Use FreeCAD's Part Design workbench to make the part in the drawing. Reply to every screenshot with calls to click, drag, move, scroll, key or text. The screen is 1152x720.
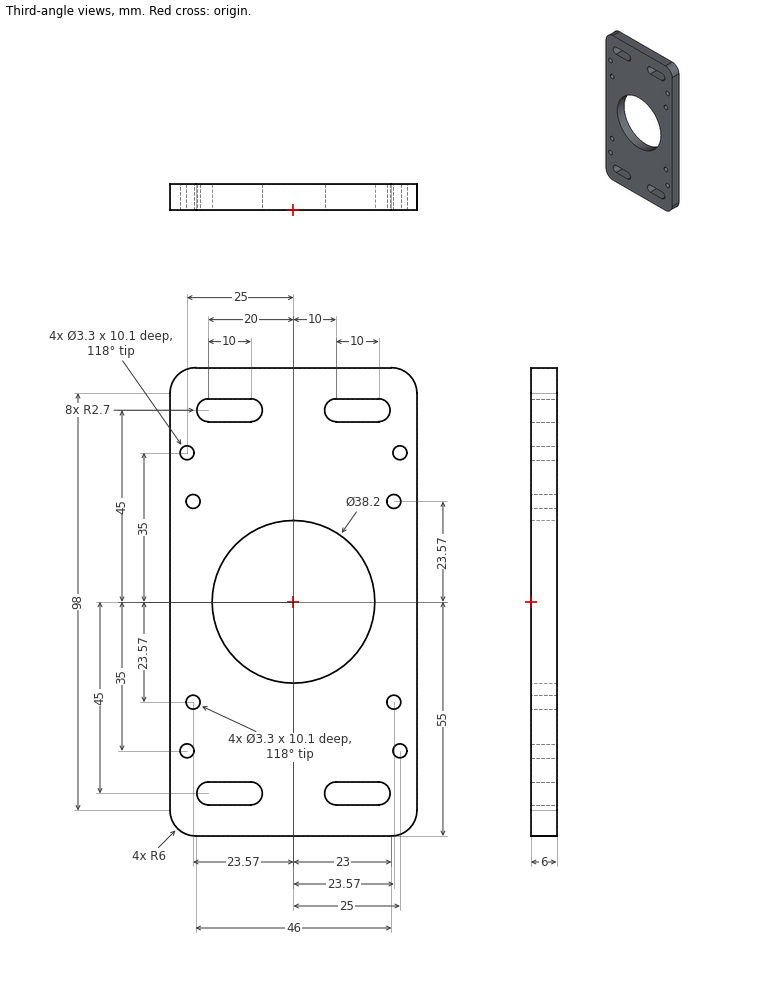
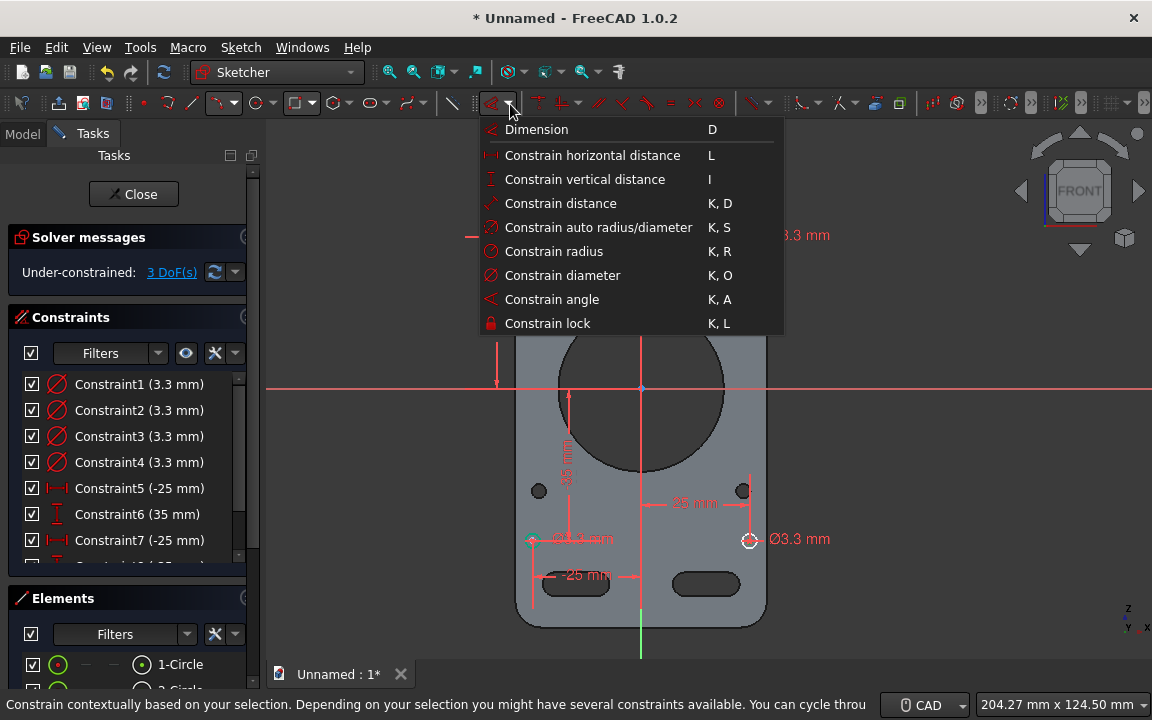
click(632, 179)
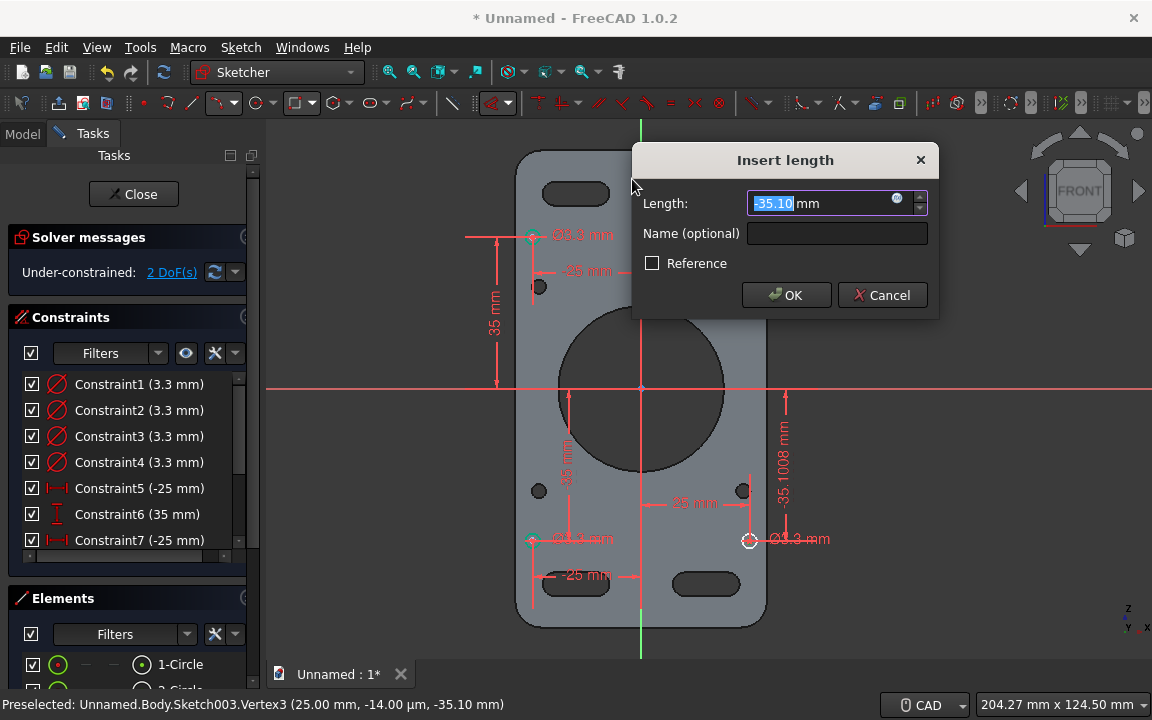
text(-35)
key(Return)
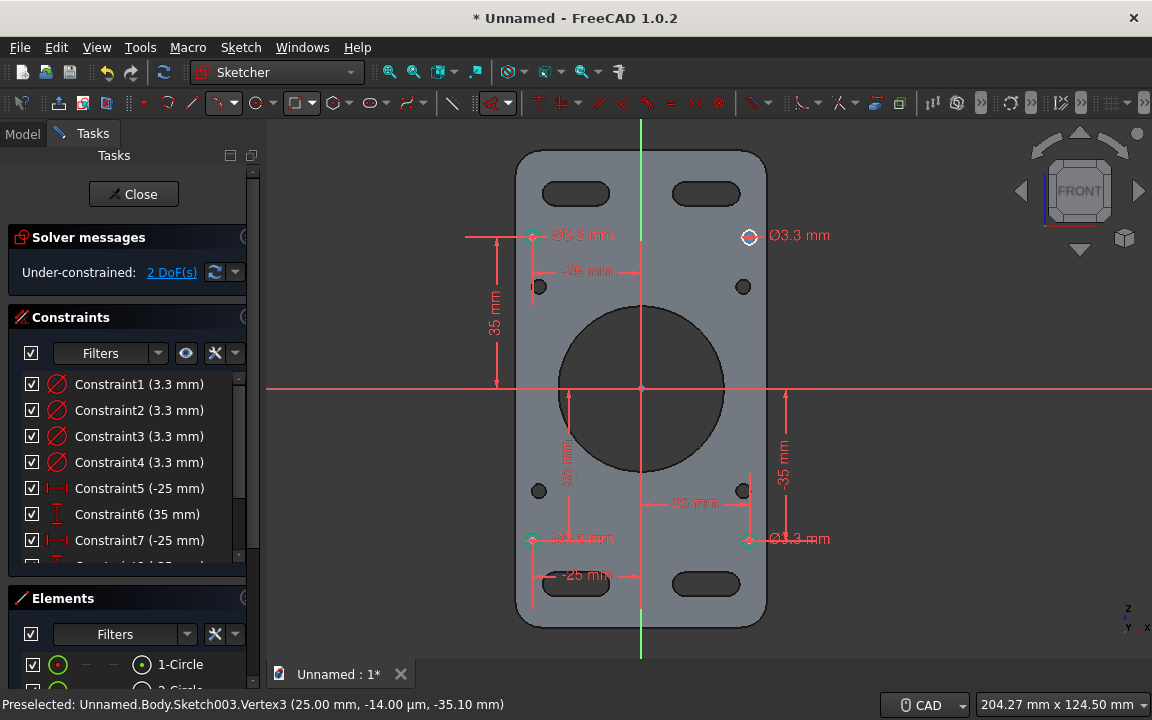
click(749, 237)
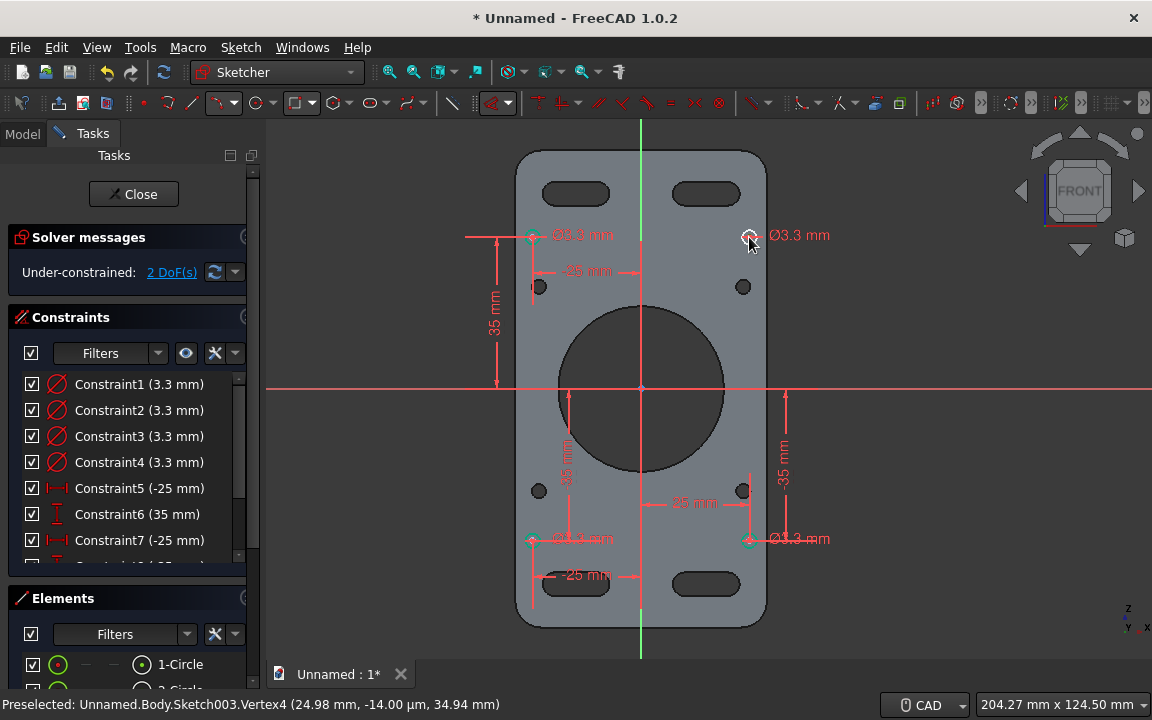
click(510, 104)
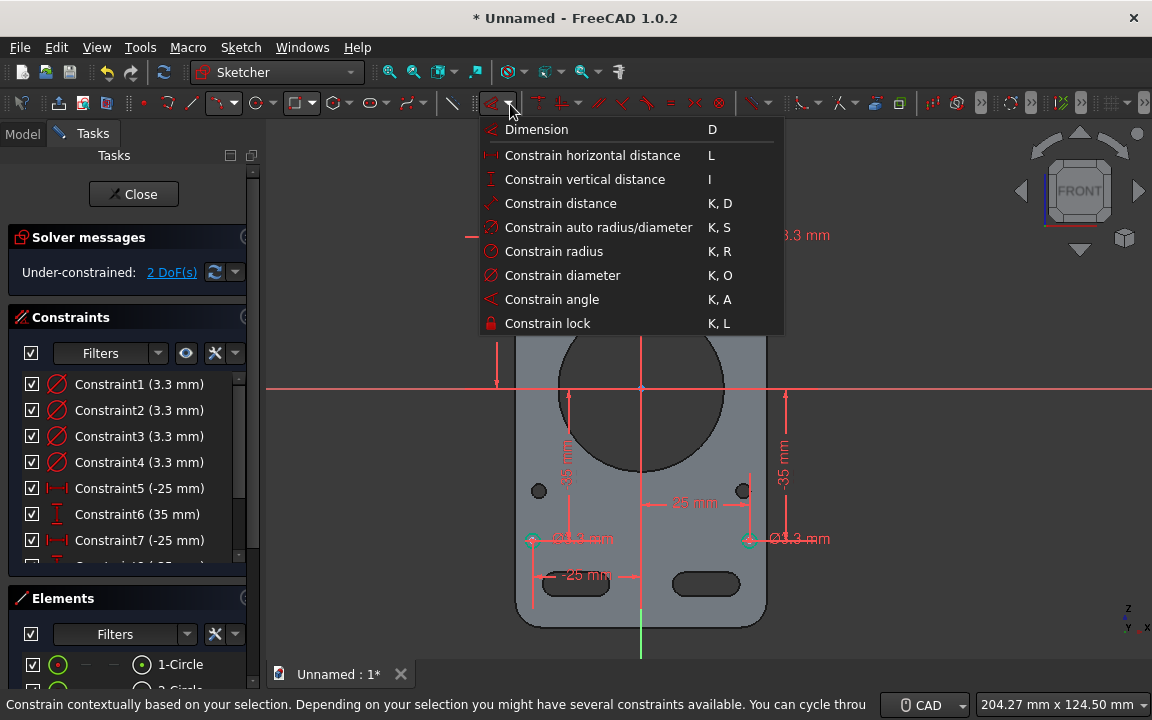
click(632, 155)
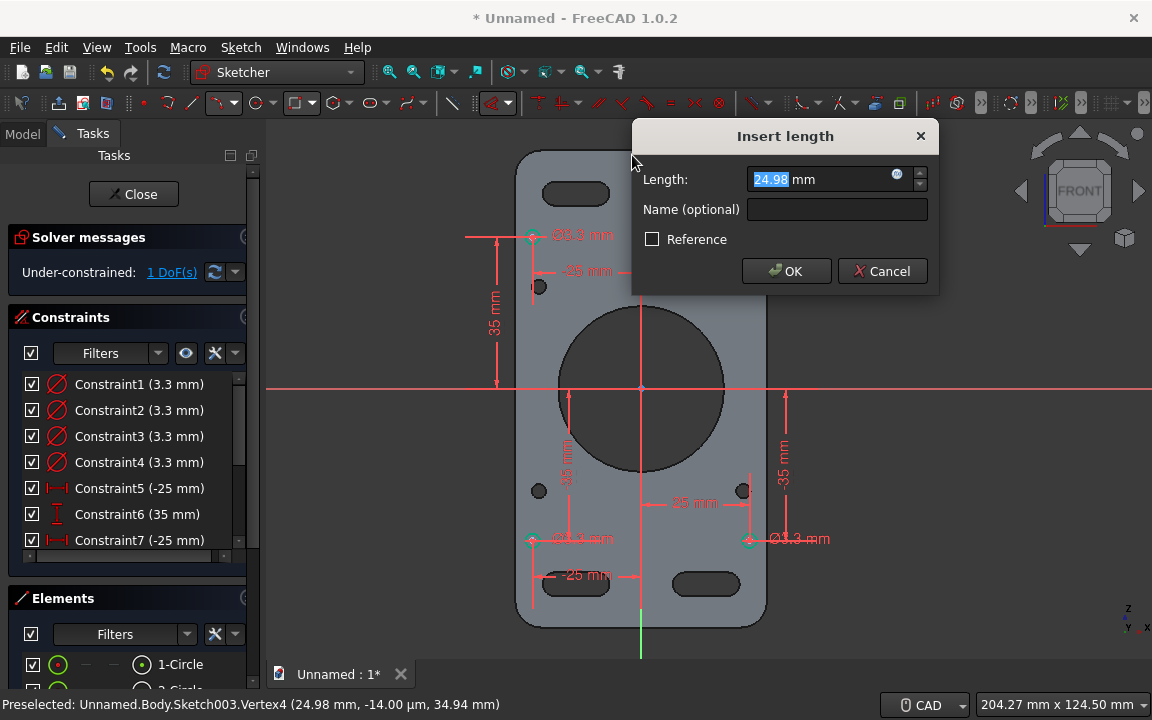
text(25)
key(Return)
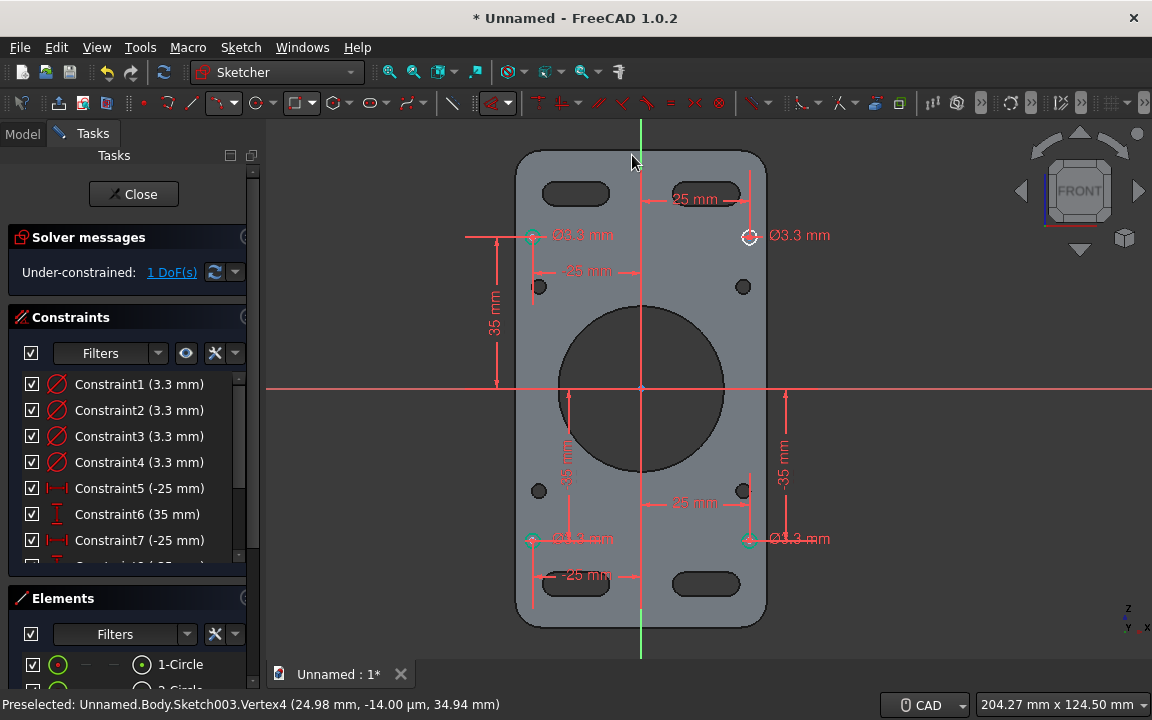
click(750, 237)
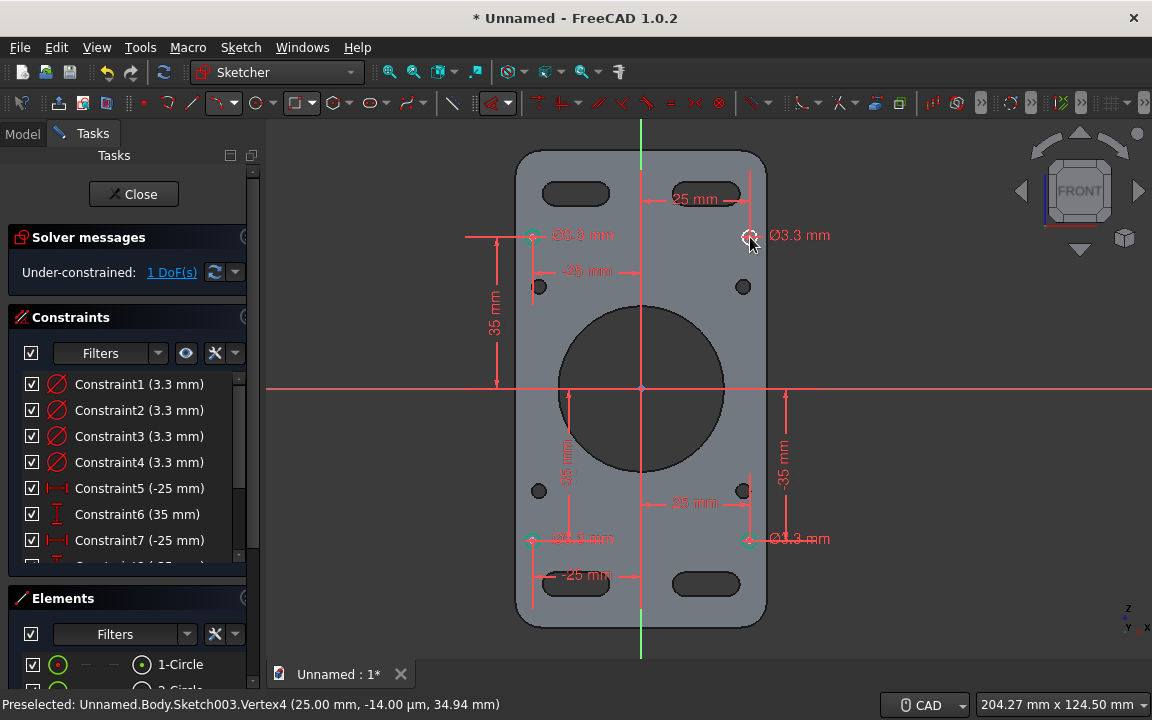
key(i)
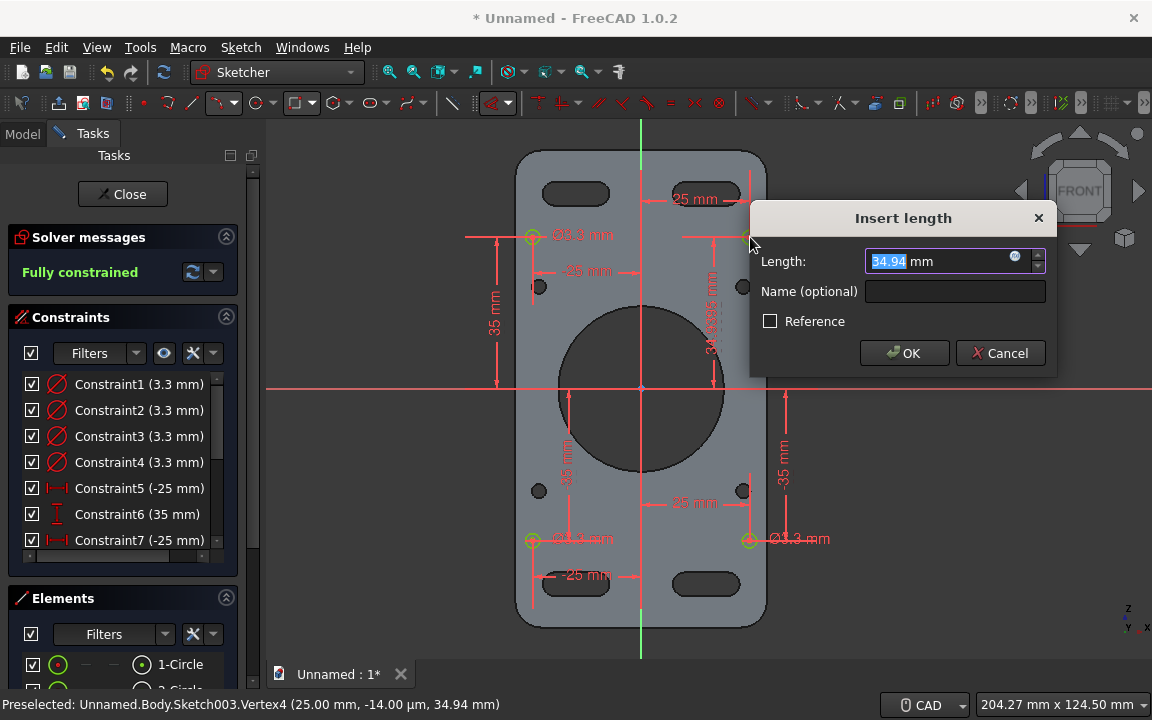
text(35)
key(Return)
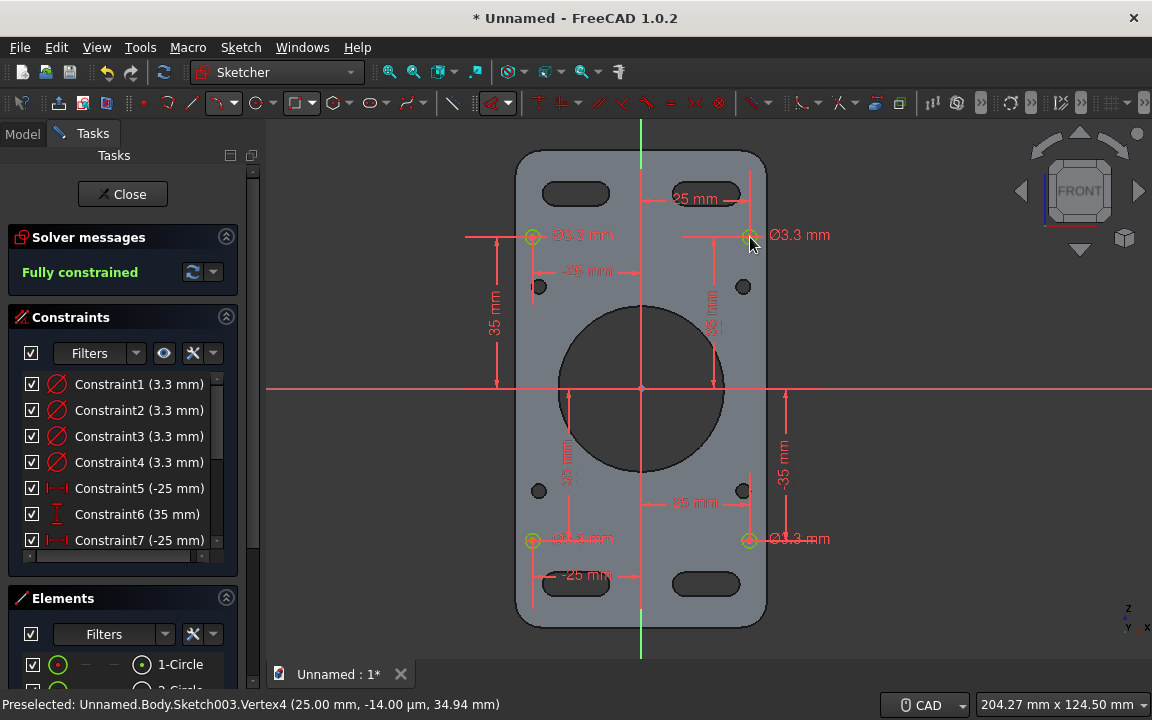
click(123, 194)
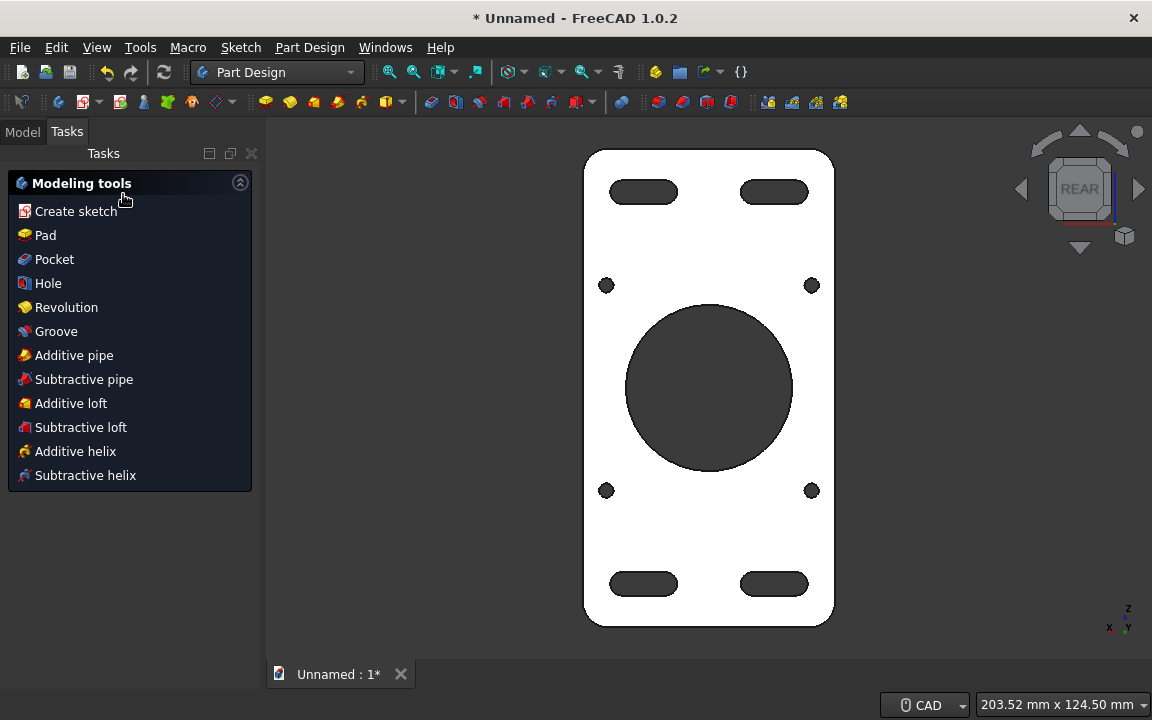
click(456, 102)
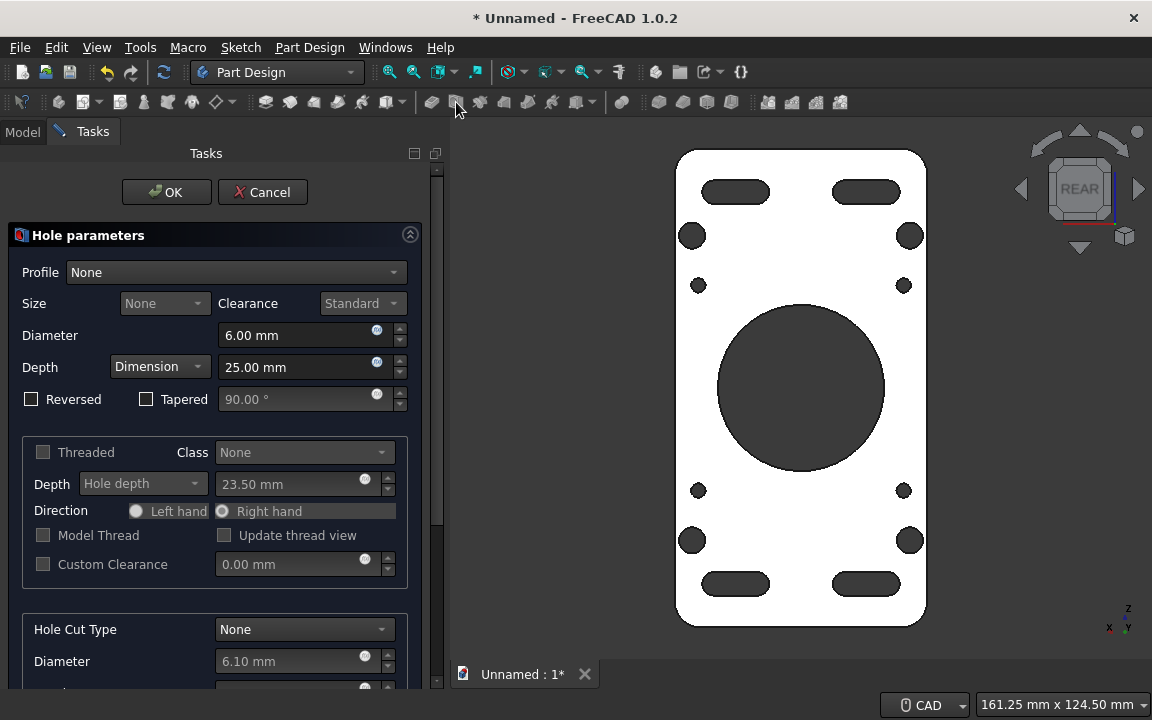
triple_click(305, 335)